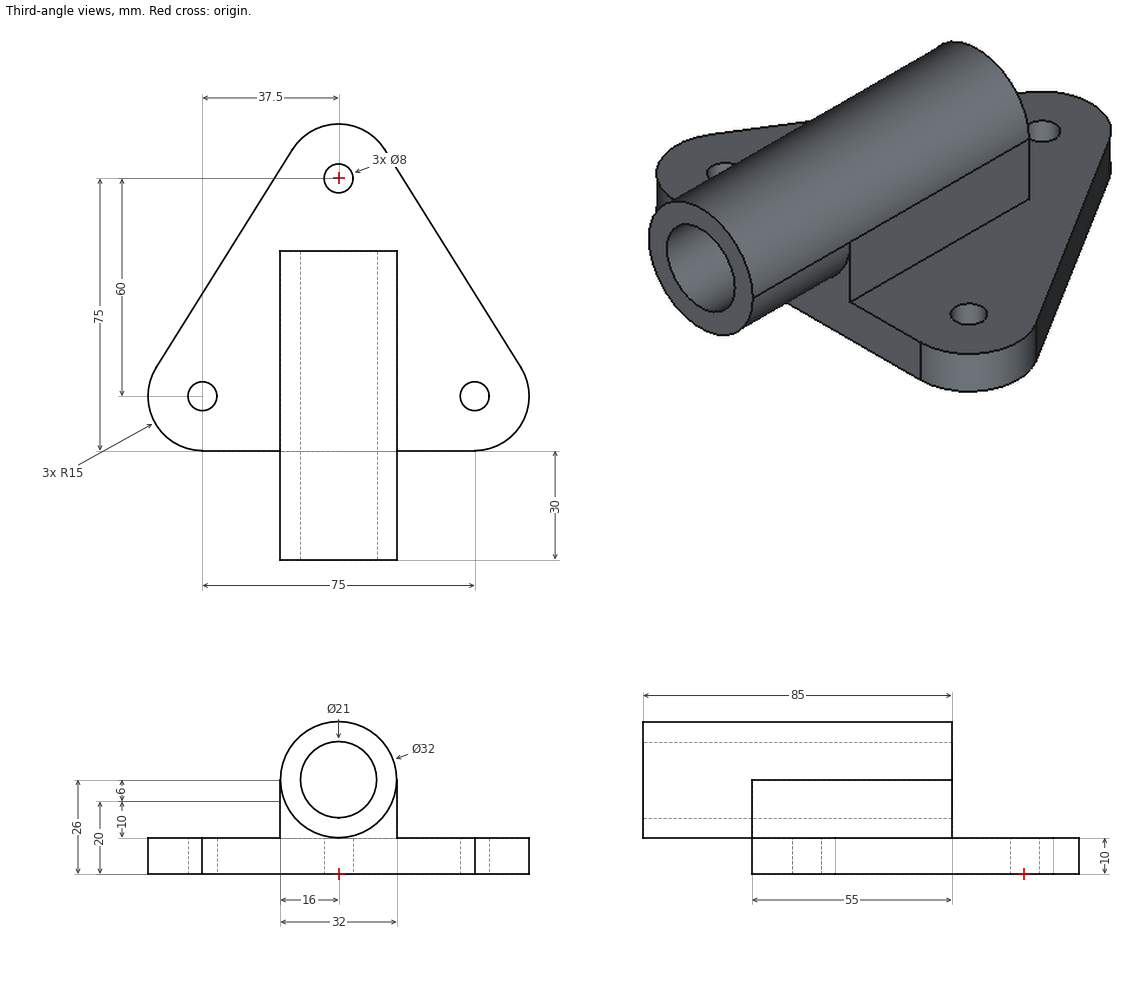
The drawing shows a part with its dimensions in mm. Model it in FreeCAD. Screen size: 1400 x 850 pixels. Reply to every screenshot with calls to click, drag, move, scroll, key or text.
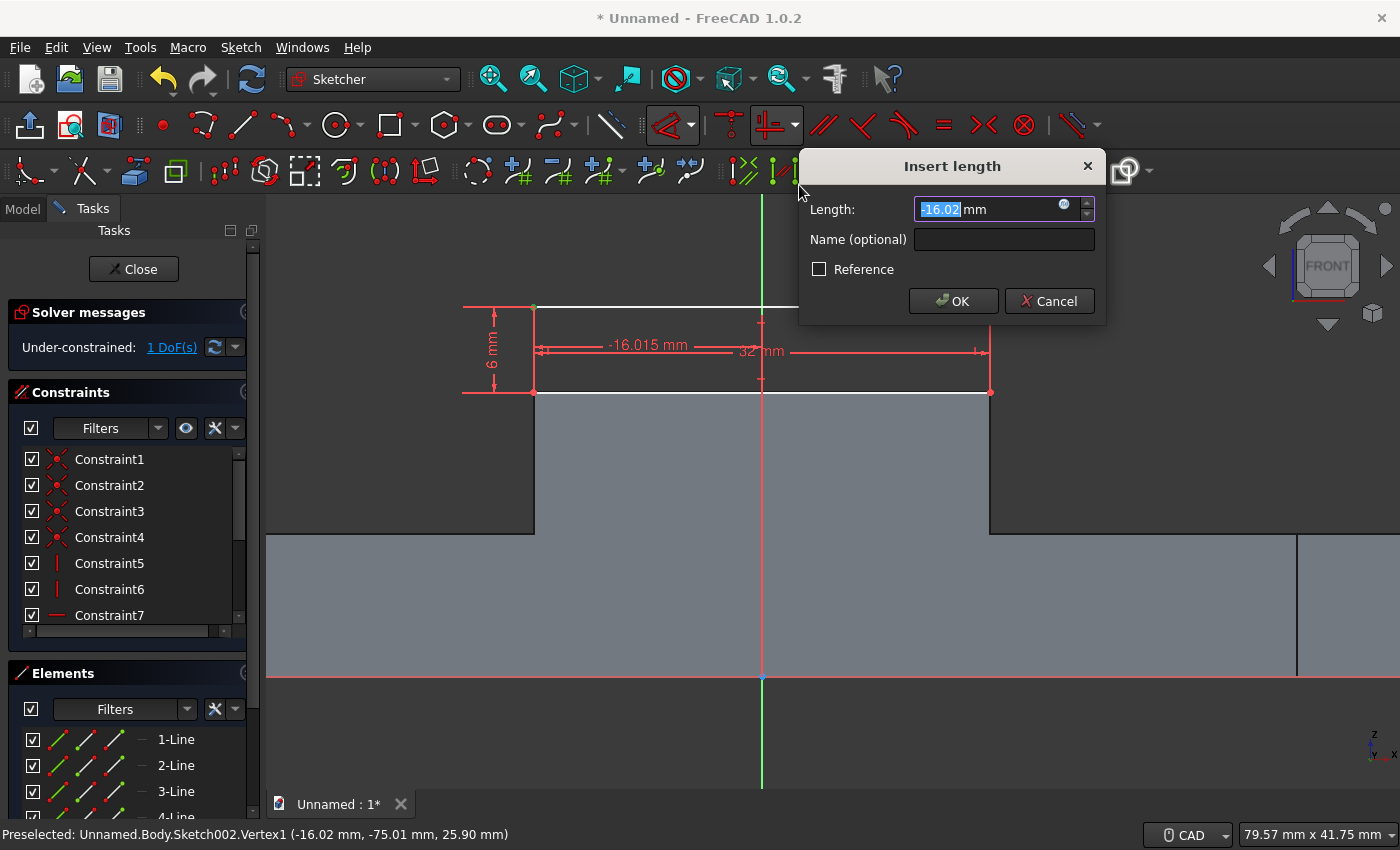
text(-16)
key(Return)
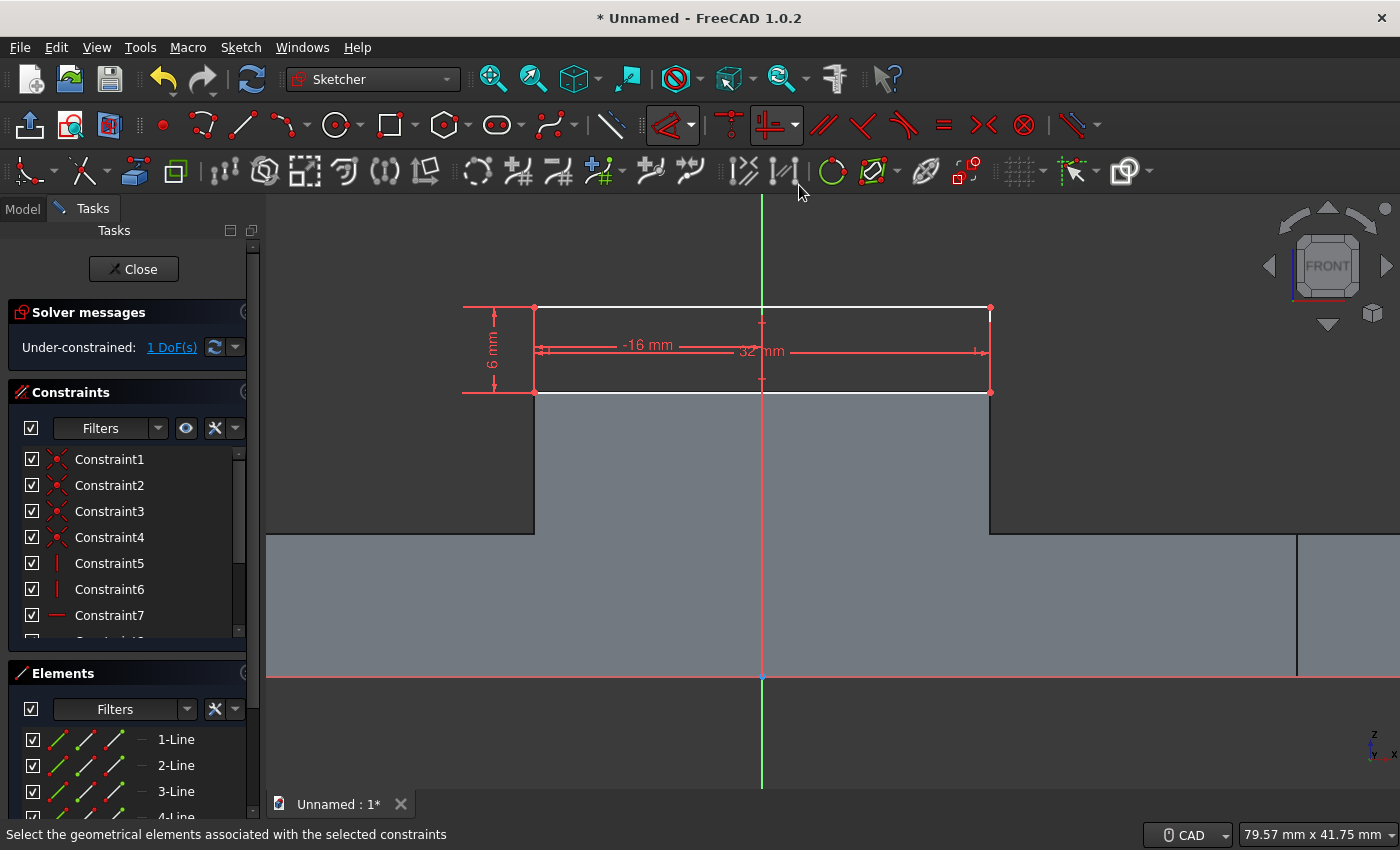
click(534, 307)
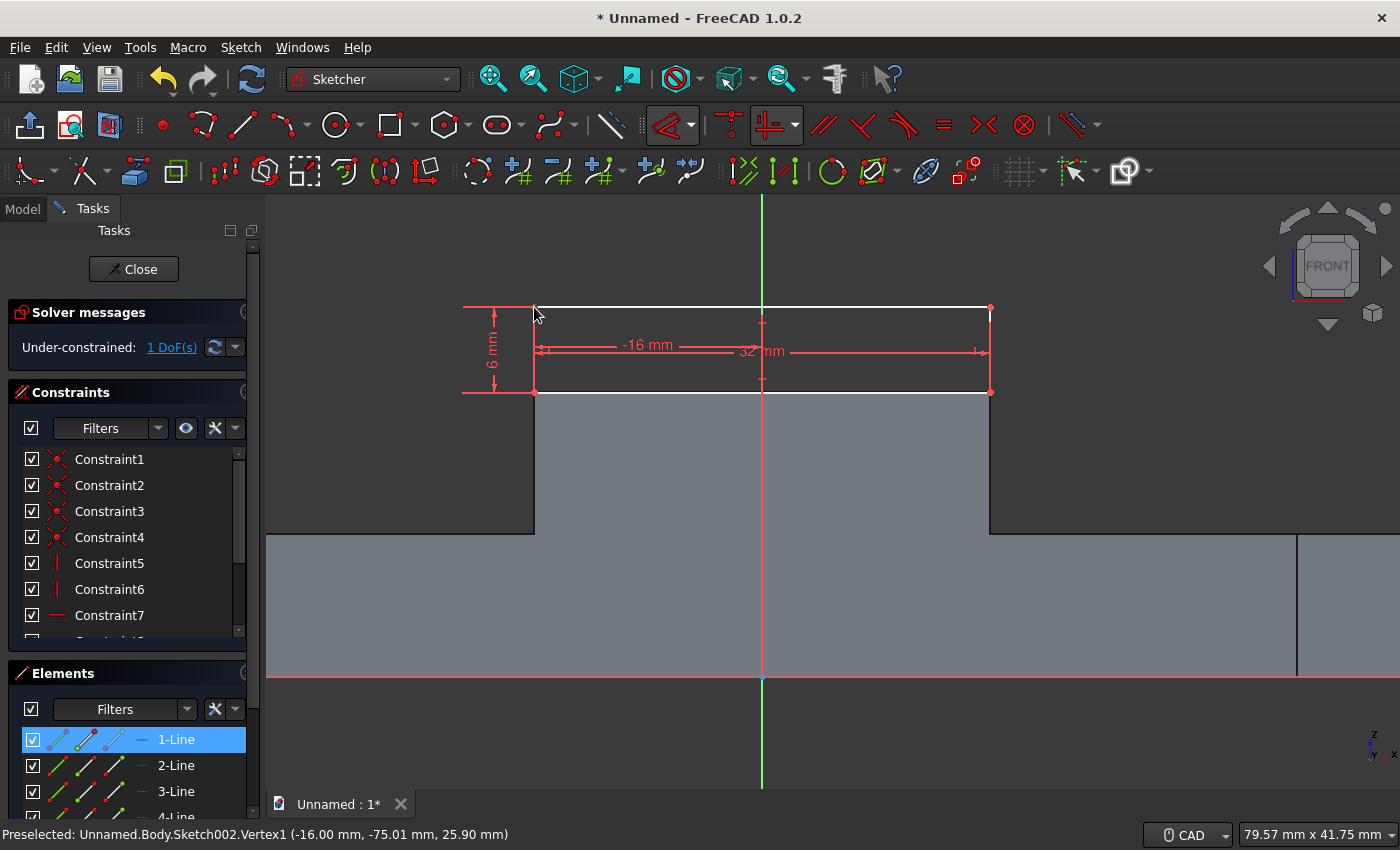
click(694, 126)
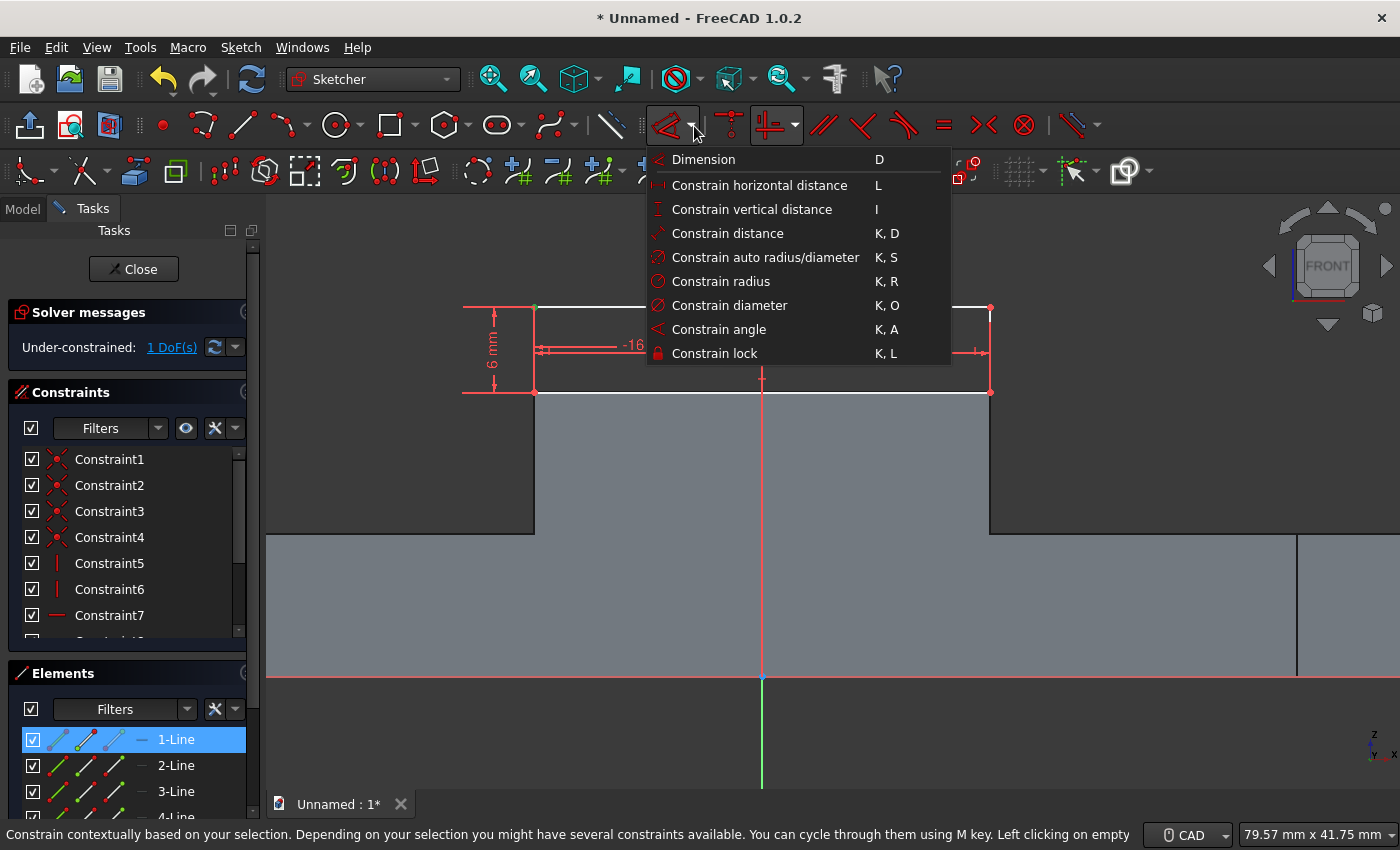
click(799, 209)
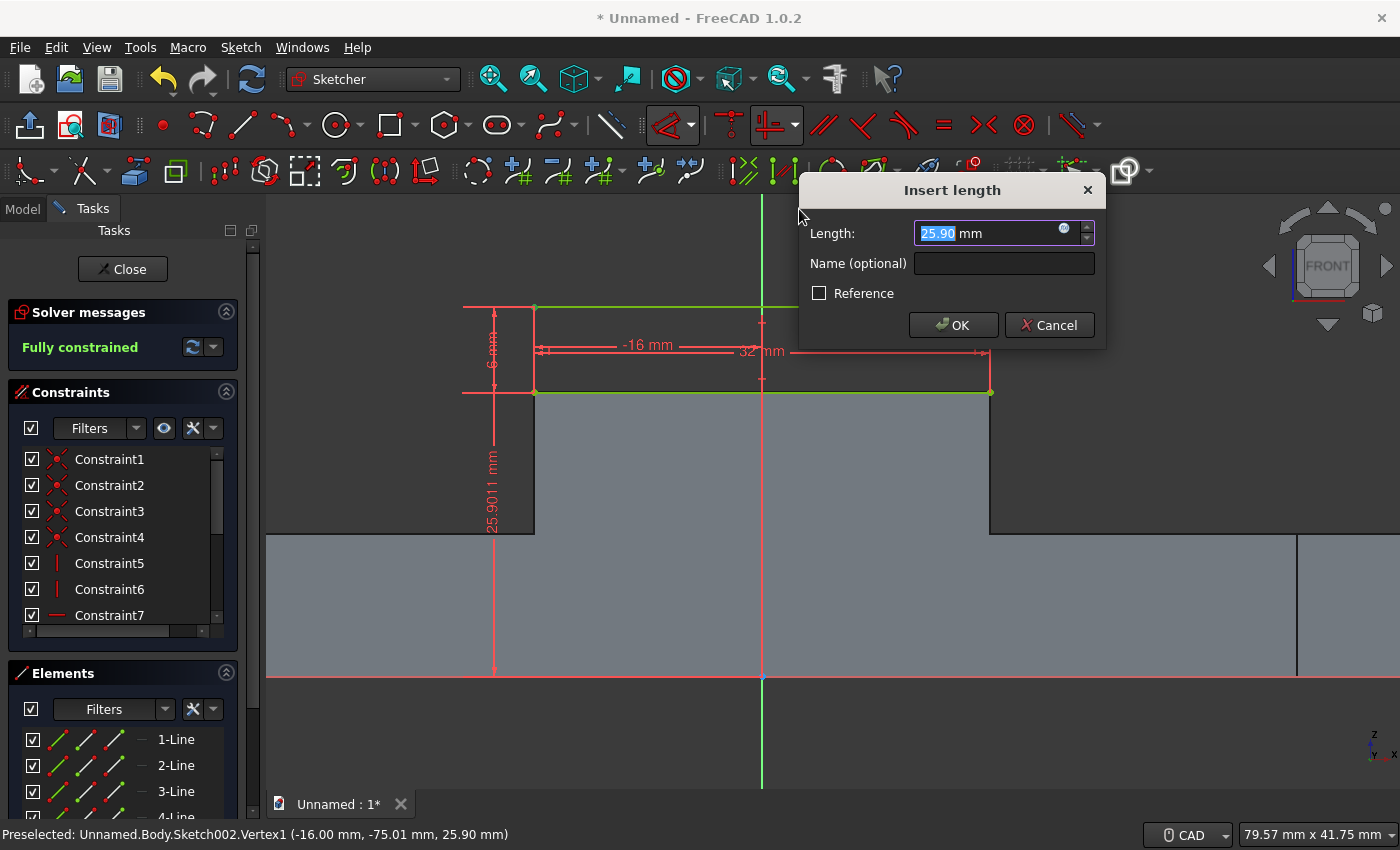
text(26)
key(Return)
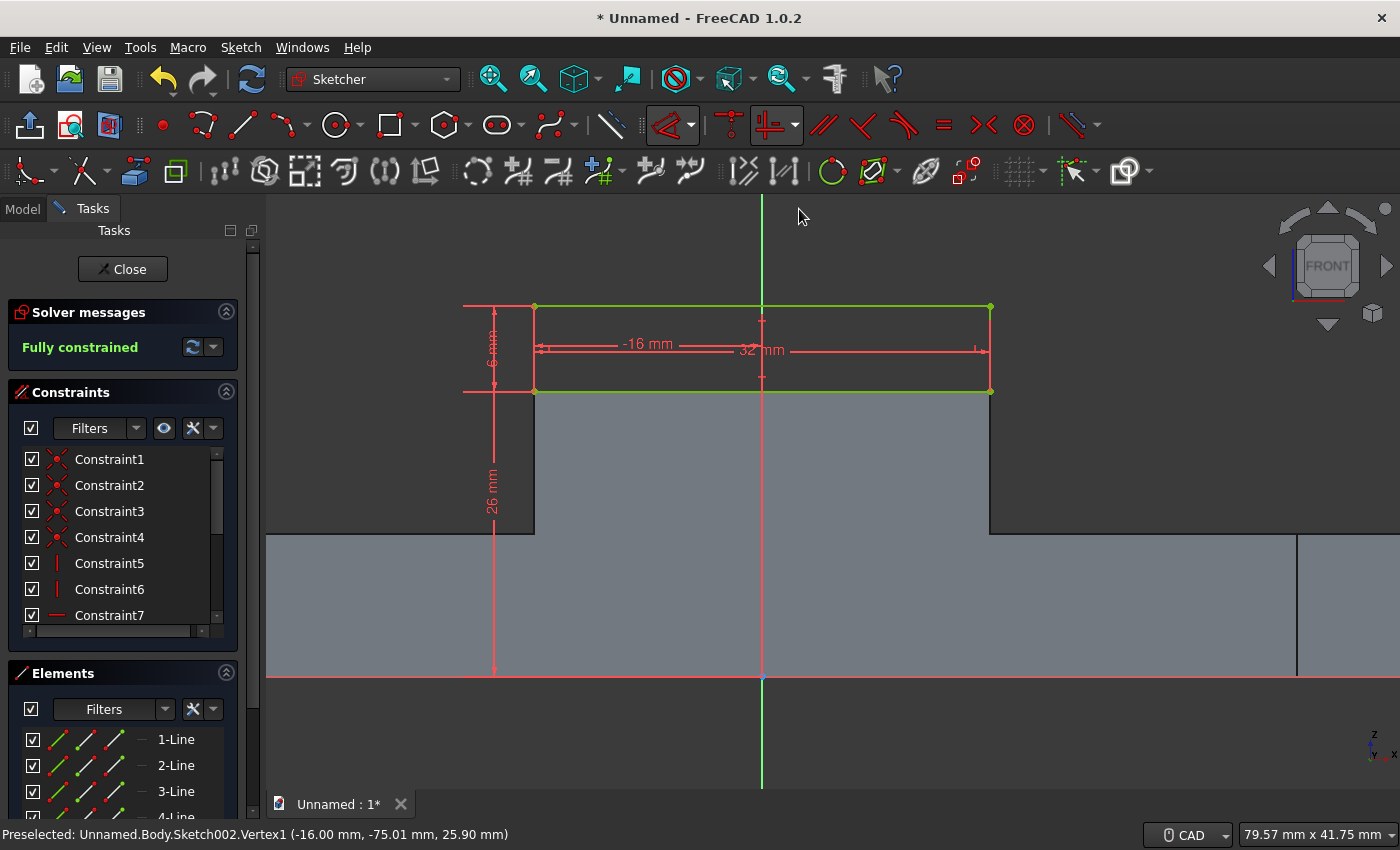
click(123, 269)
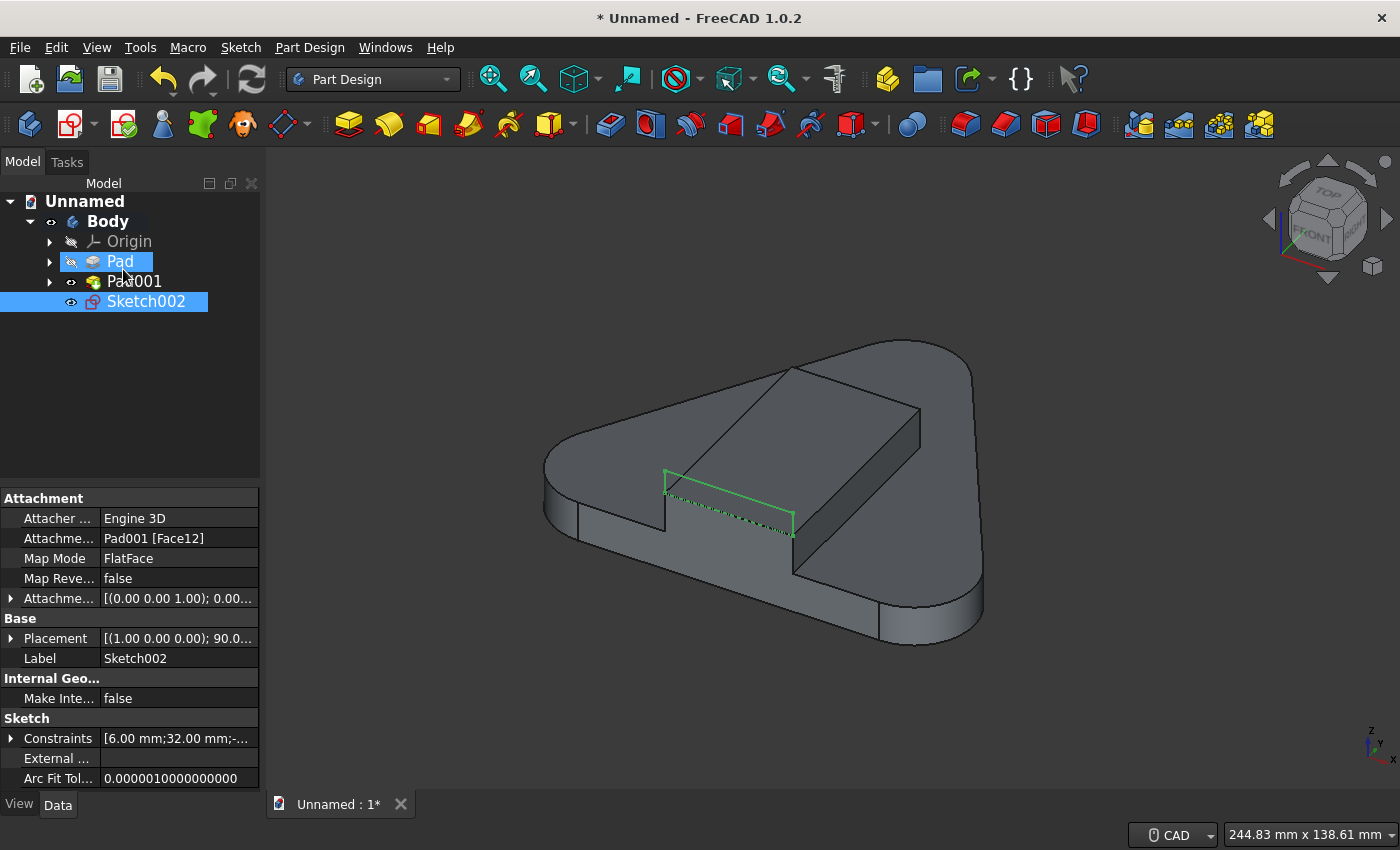
click(350, 124)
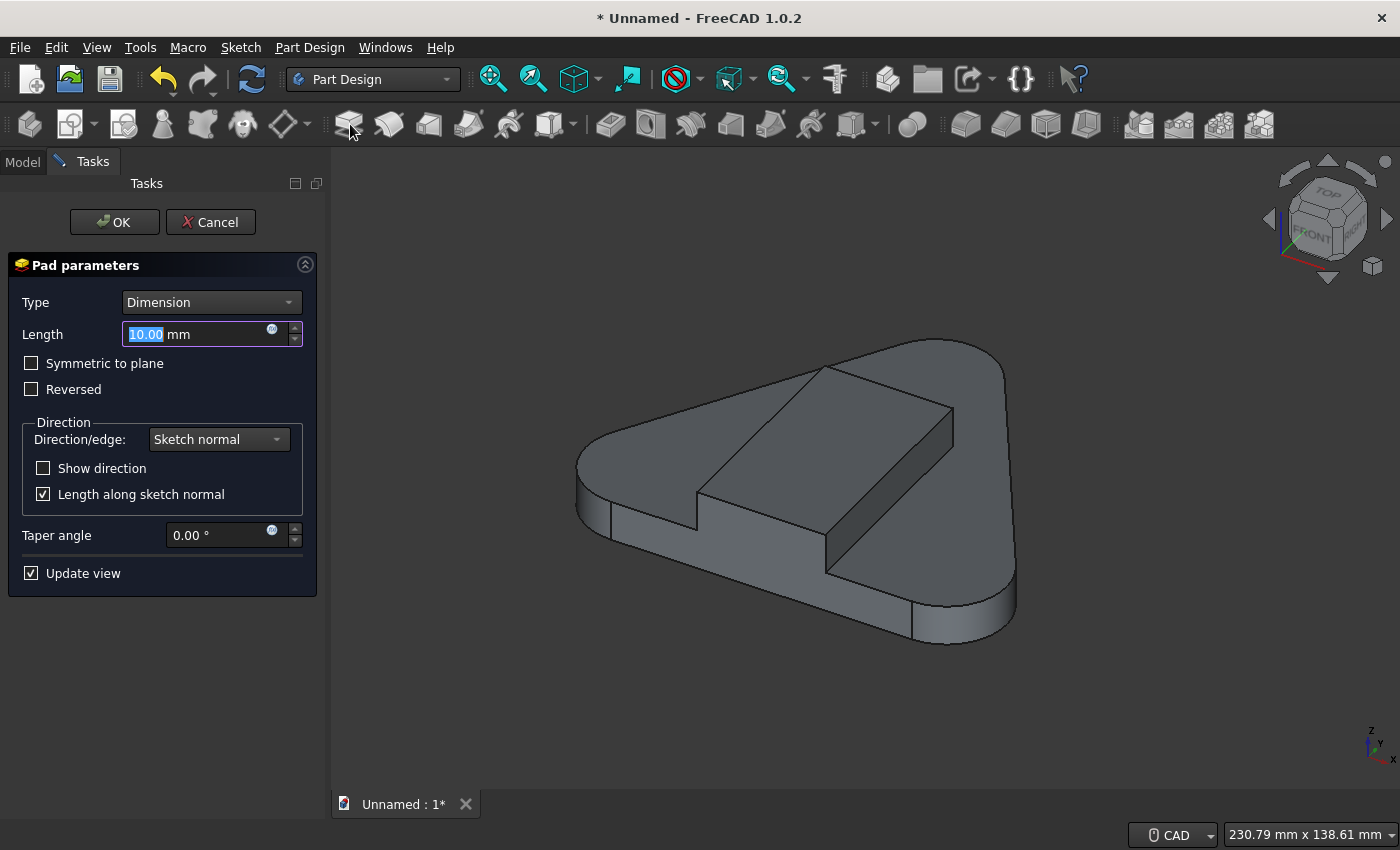
text(55)
key(Tab)